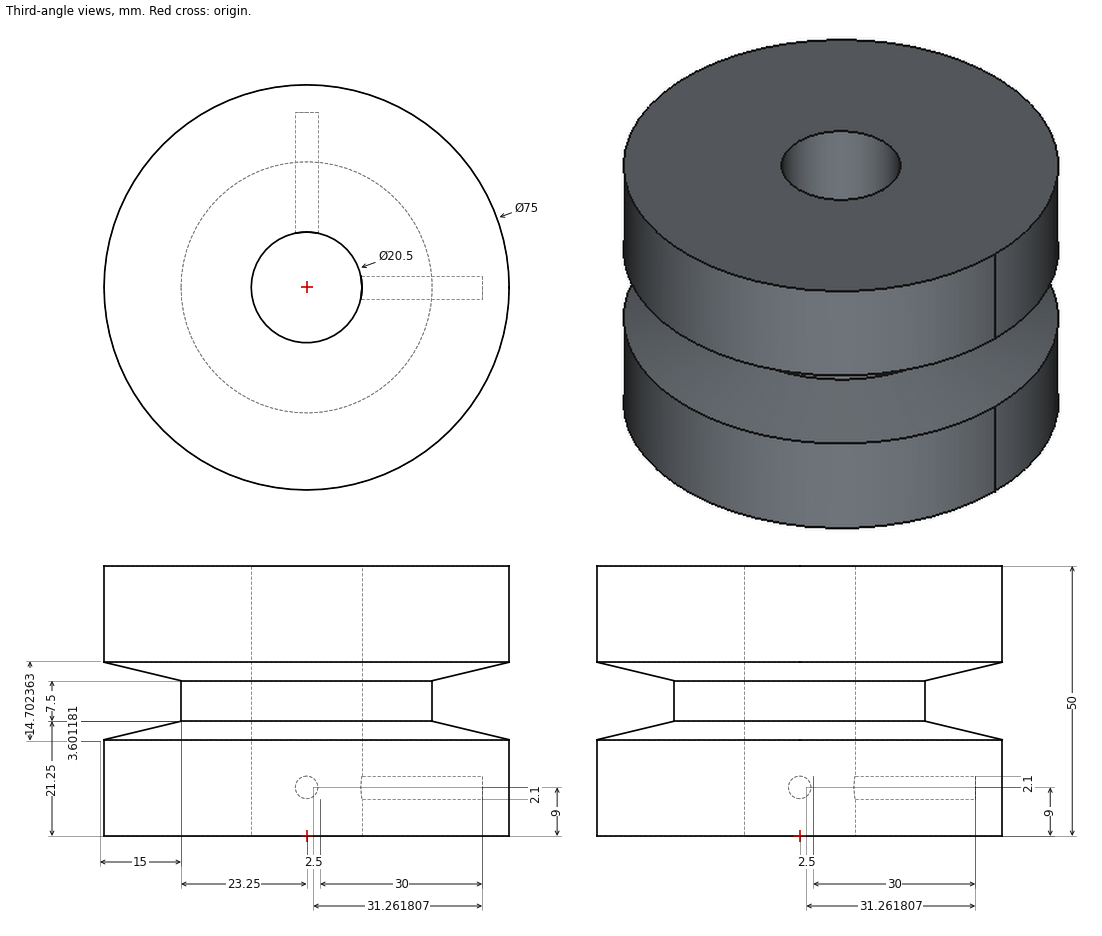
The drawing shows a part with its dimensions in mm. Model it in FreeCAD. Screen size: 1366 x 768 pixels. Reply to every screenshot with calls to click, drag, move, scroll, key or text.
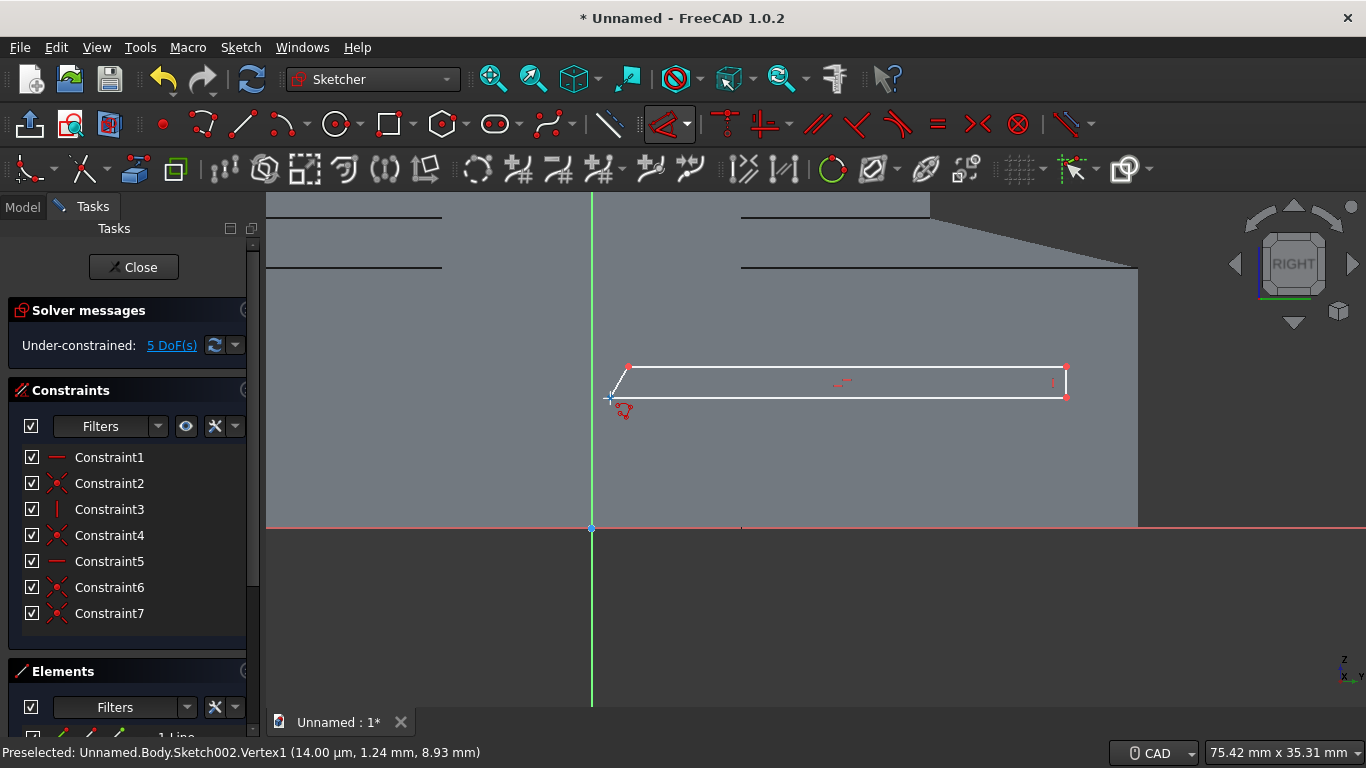
key(g)
key(l)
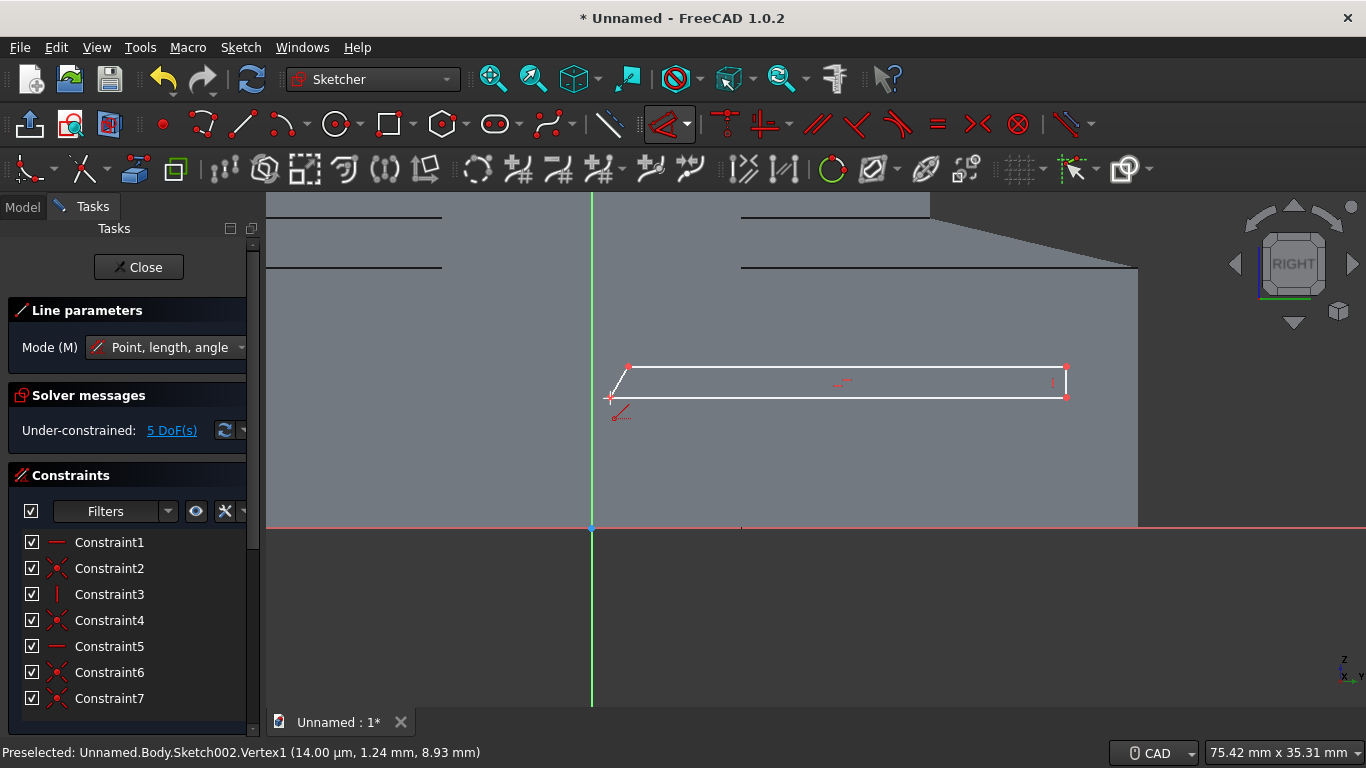
click(564, 397)
click(428, 397)
key(Escape)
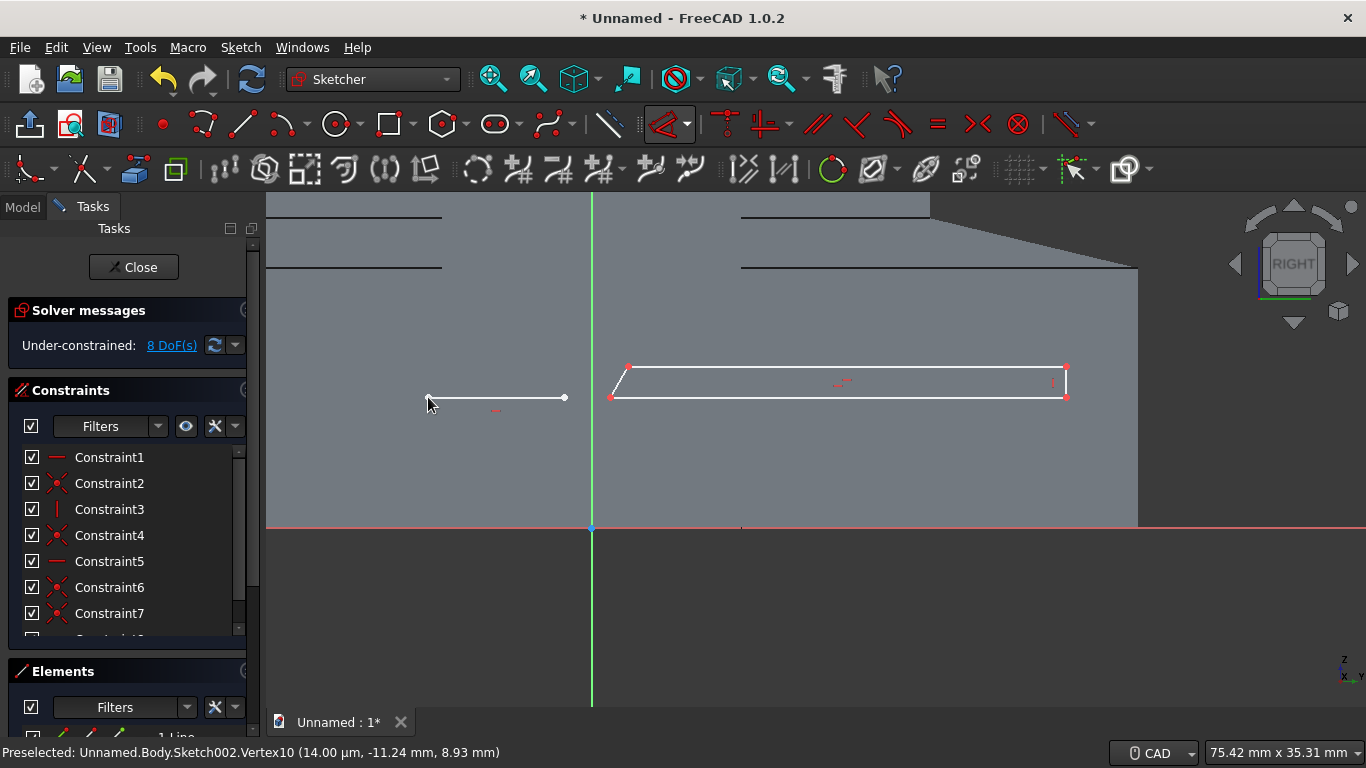
click(523, 398)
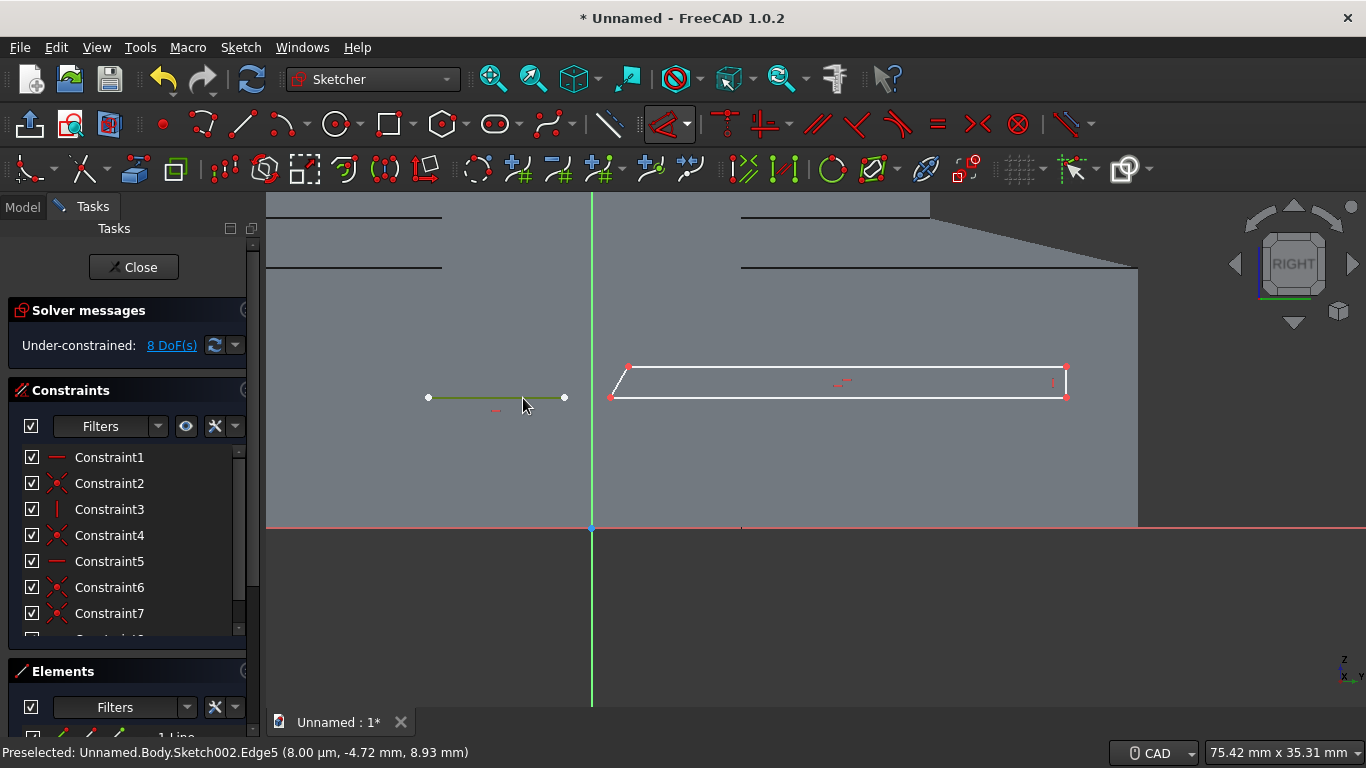
click(610, 124)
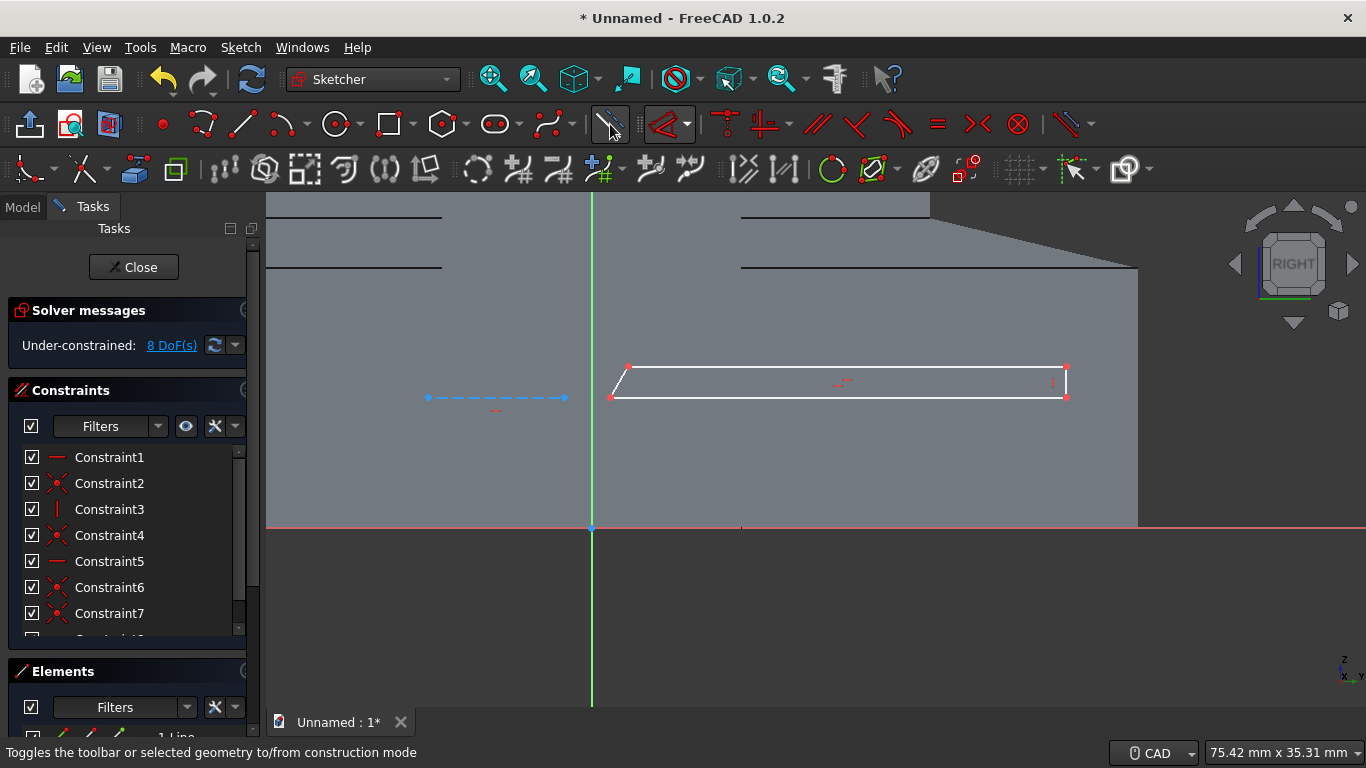
click(664, 124)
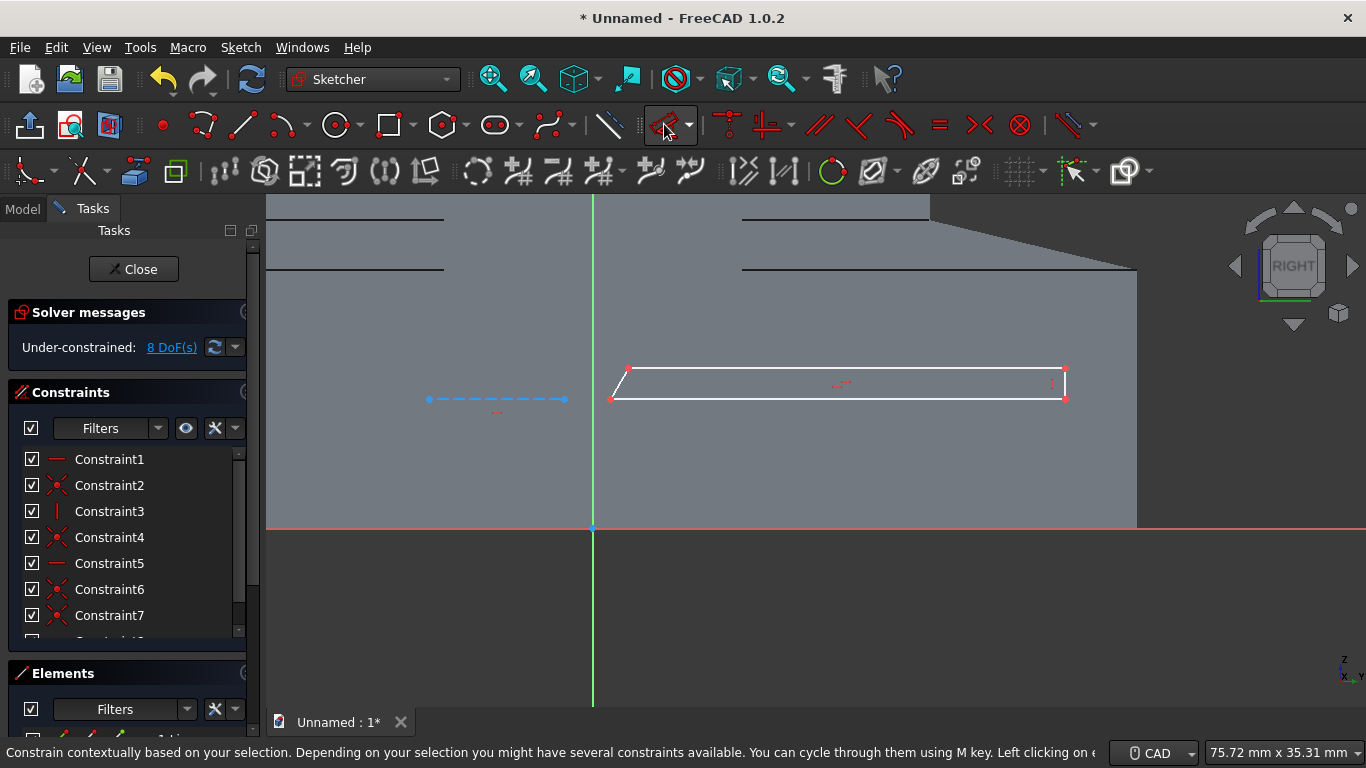
click(934, 368)
click(847, 334)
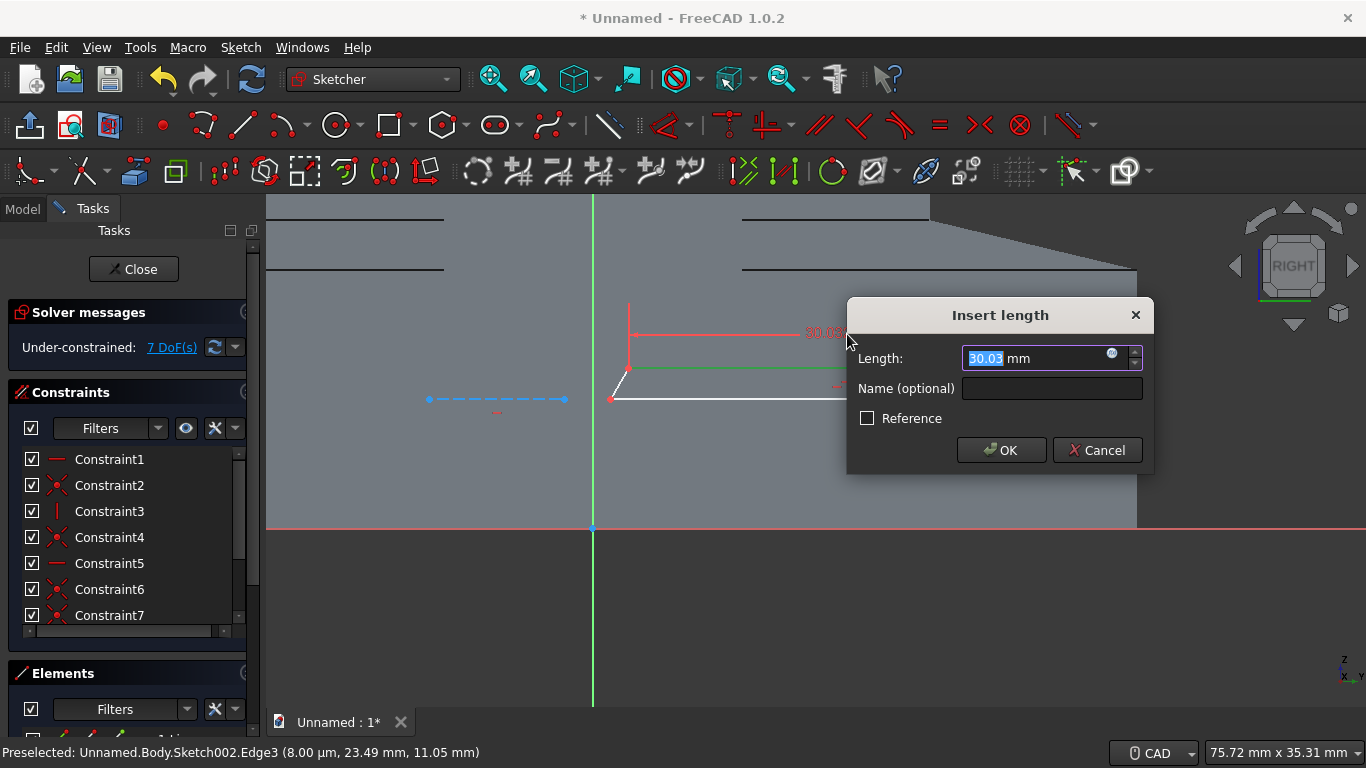
text(30)
key(Return)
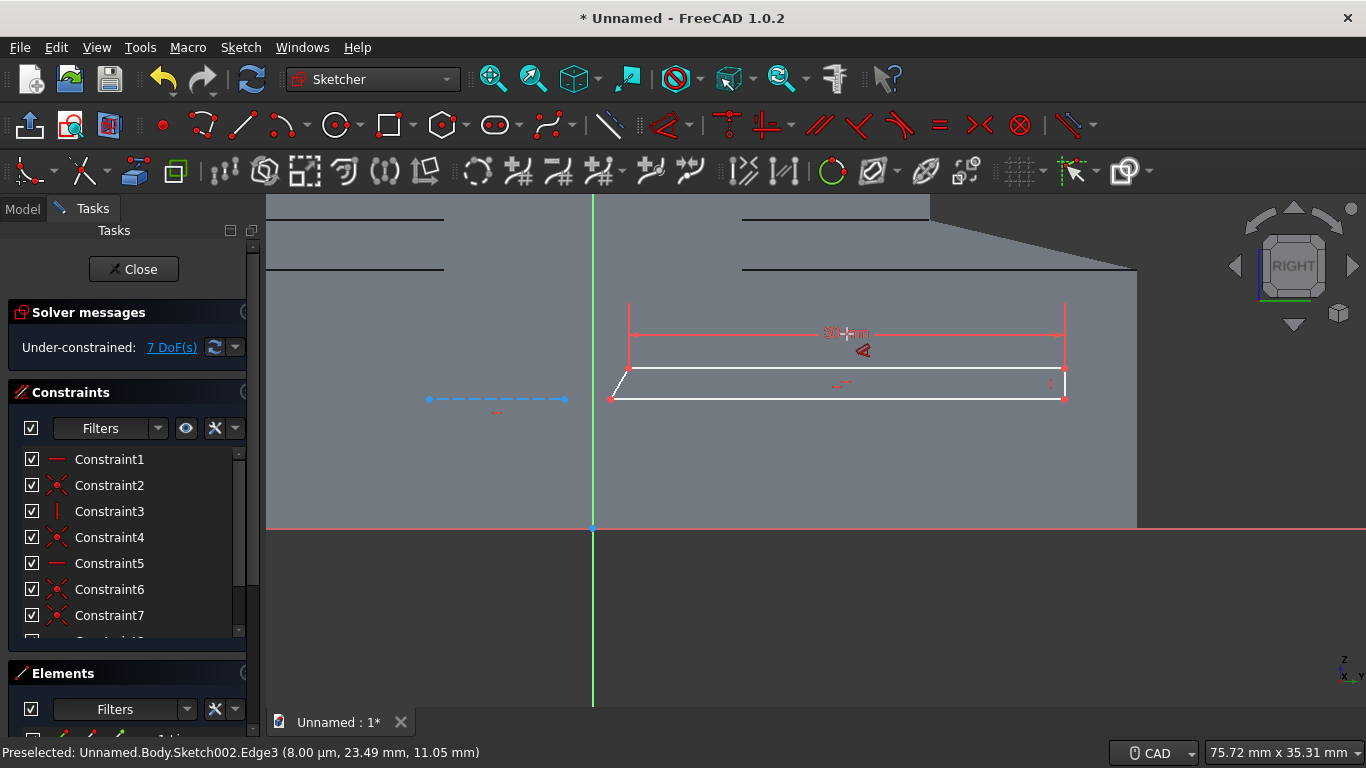
click(611, 399)
click(559, 464)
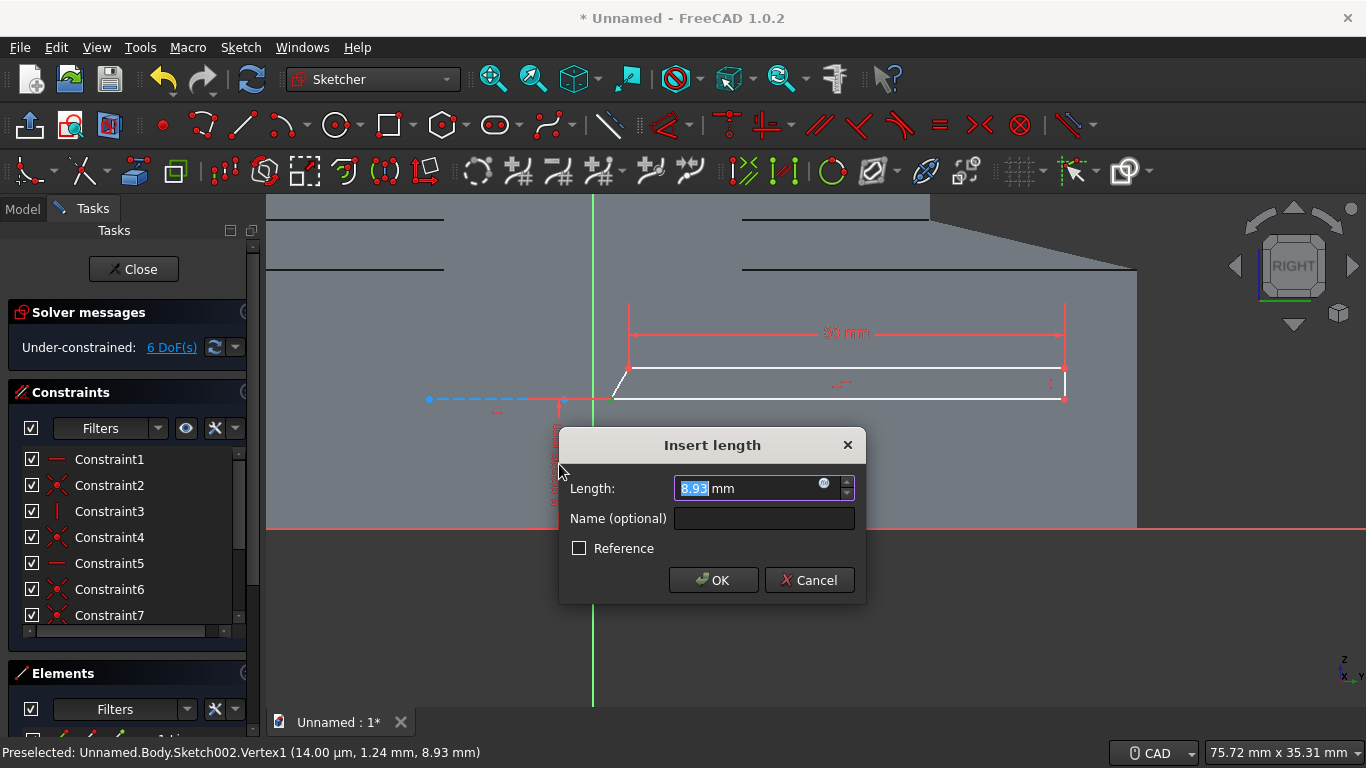
text(9)
key(Return)